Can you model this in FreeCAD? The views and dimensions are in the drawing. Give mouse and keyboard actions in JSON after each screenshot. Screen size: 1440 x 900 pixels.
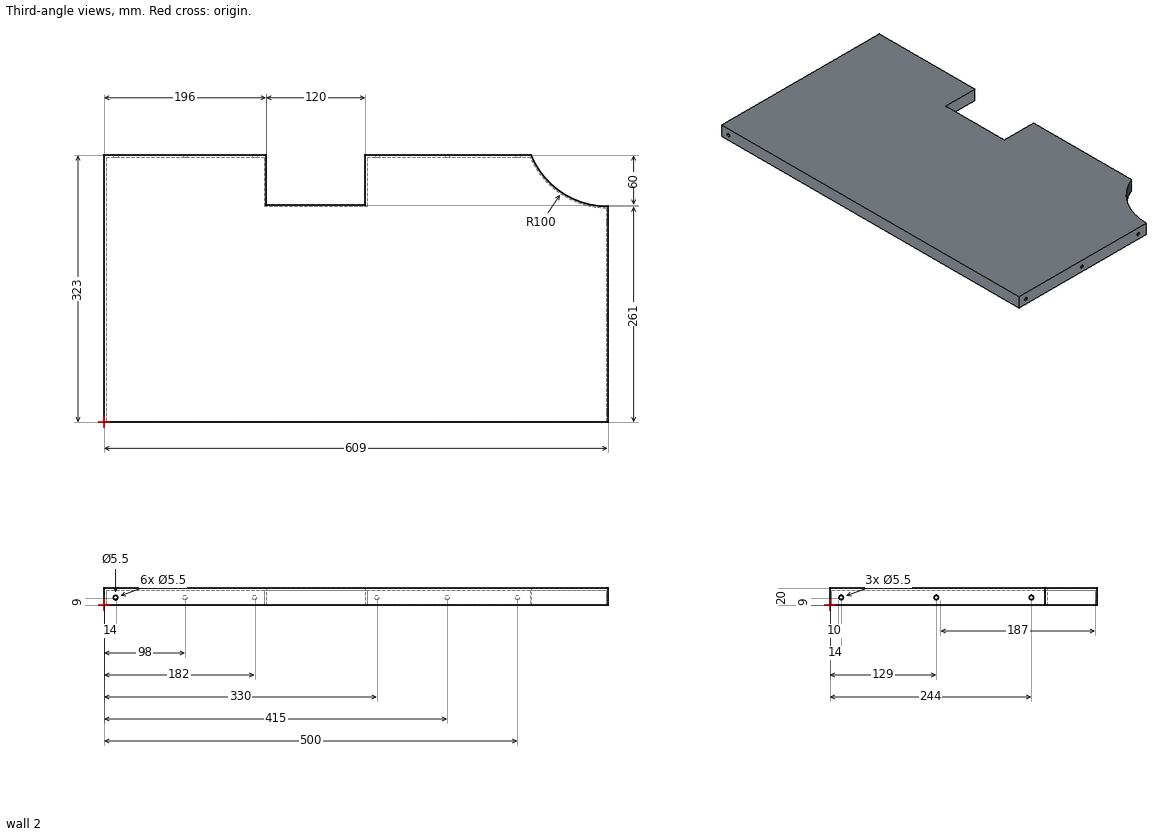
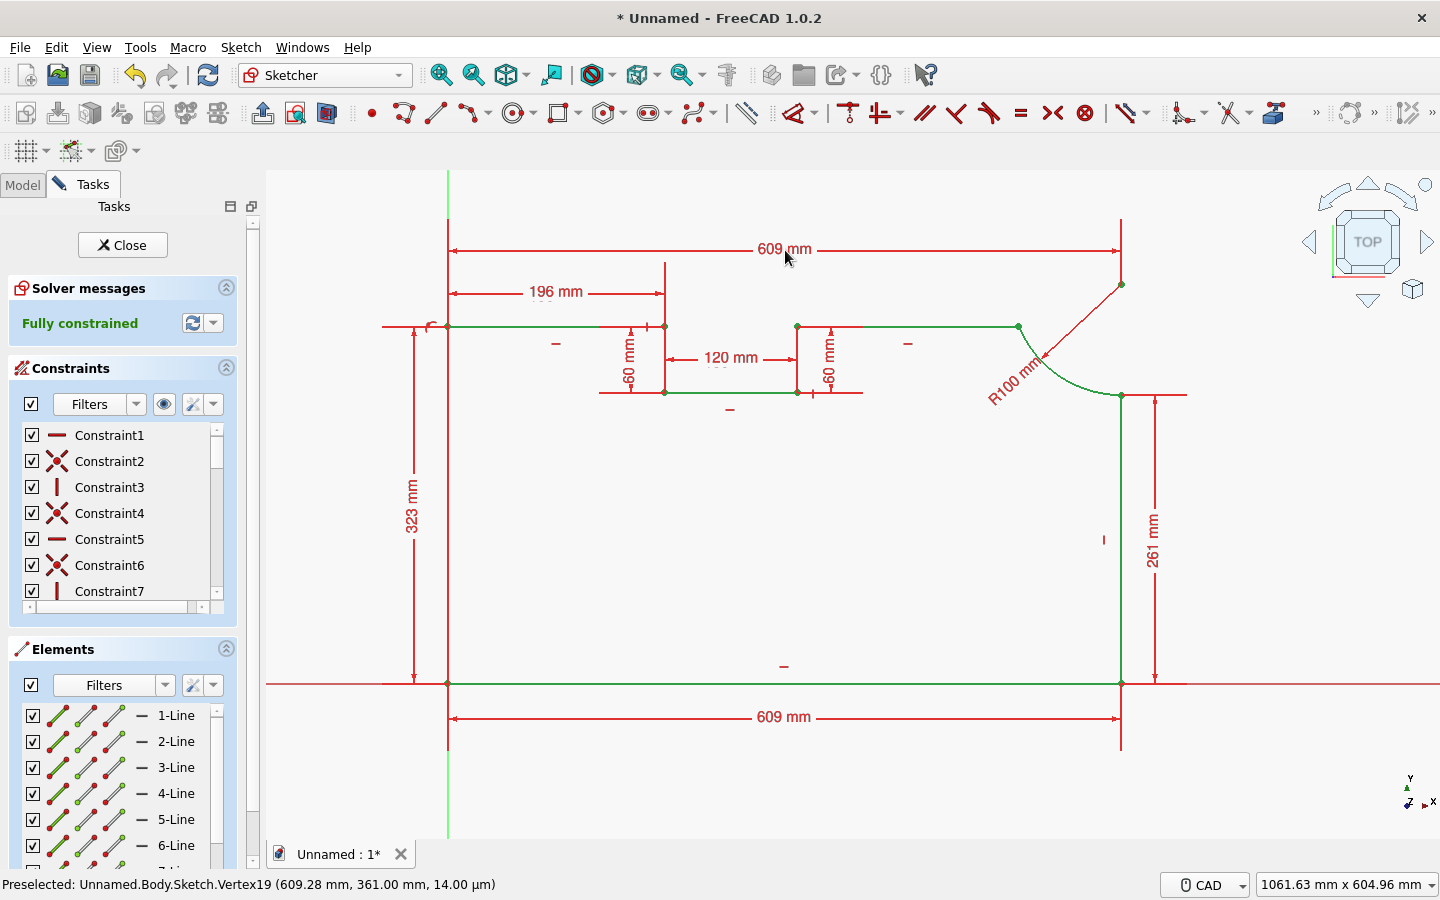
{"action": "left_click", "coordinate": [123, 245]}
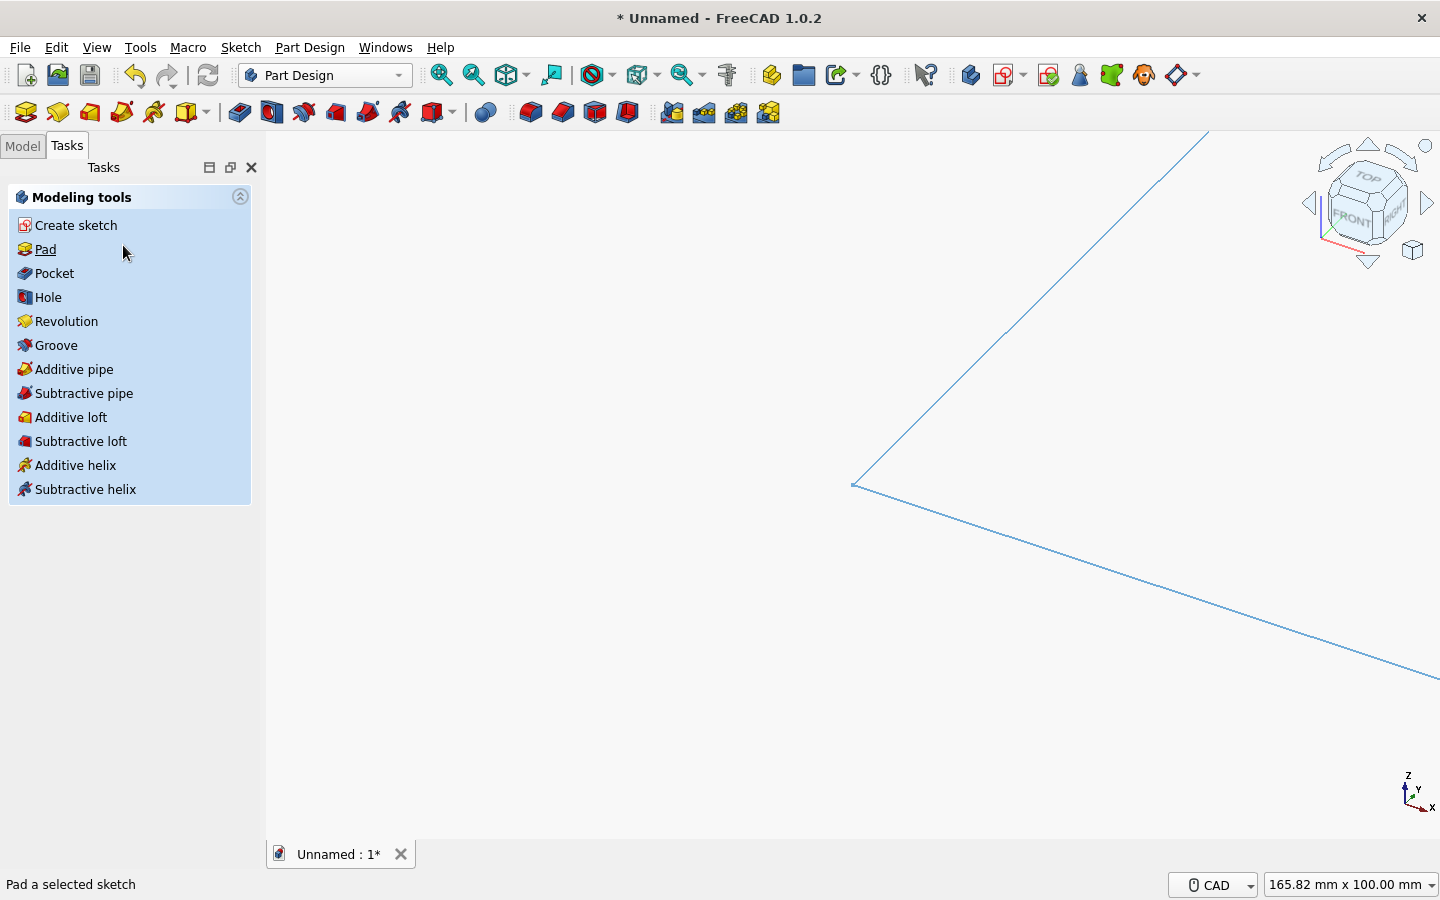
{"action": "left_click", "coordinate": [26, 112]}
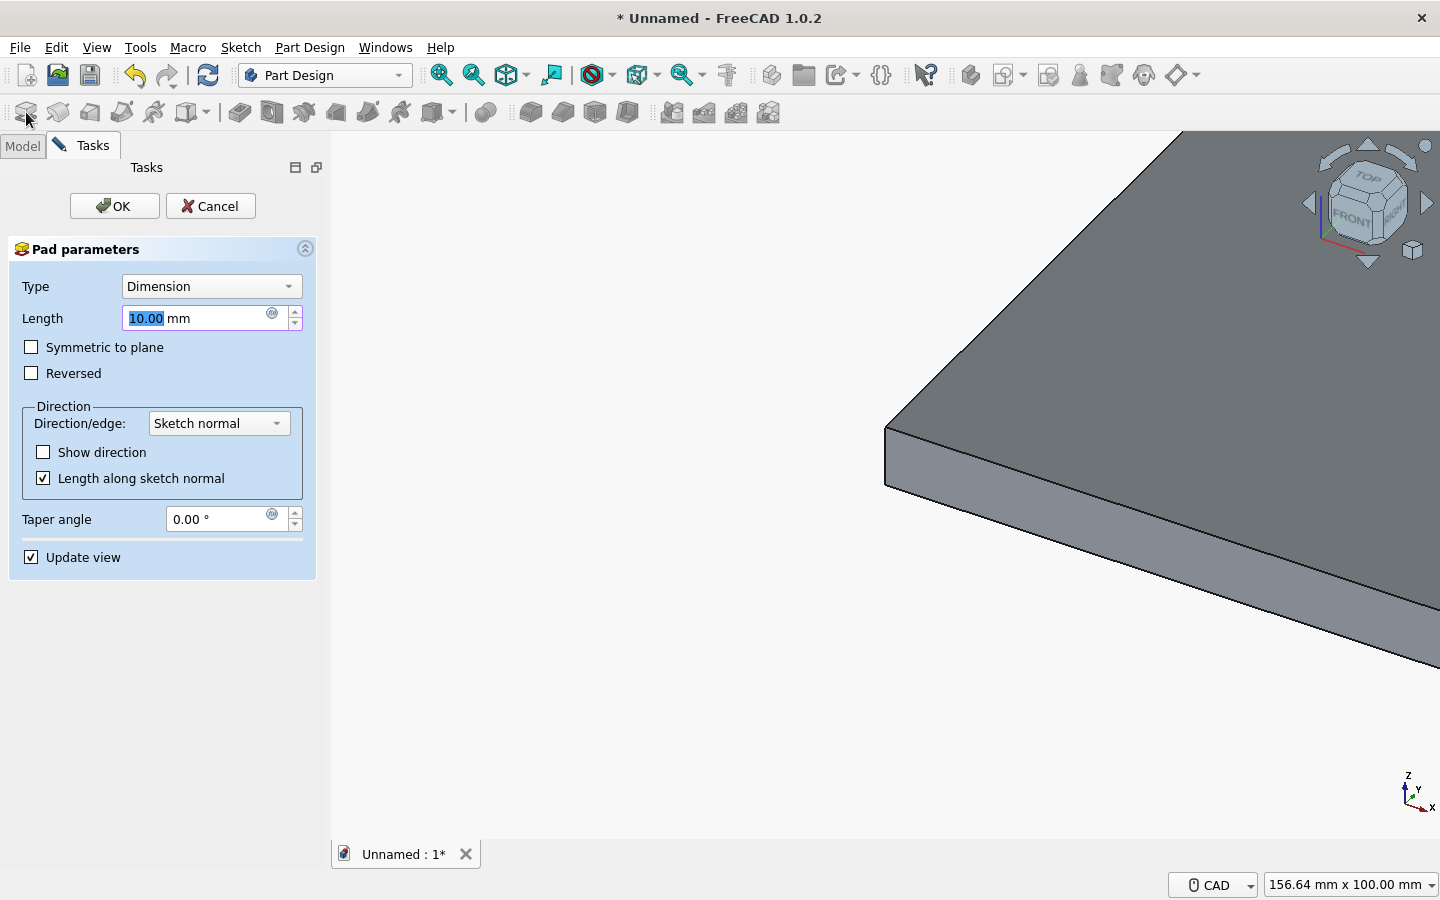
{"action": "type", "text": "20"}
{"action": "key", "text": "Tab"}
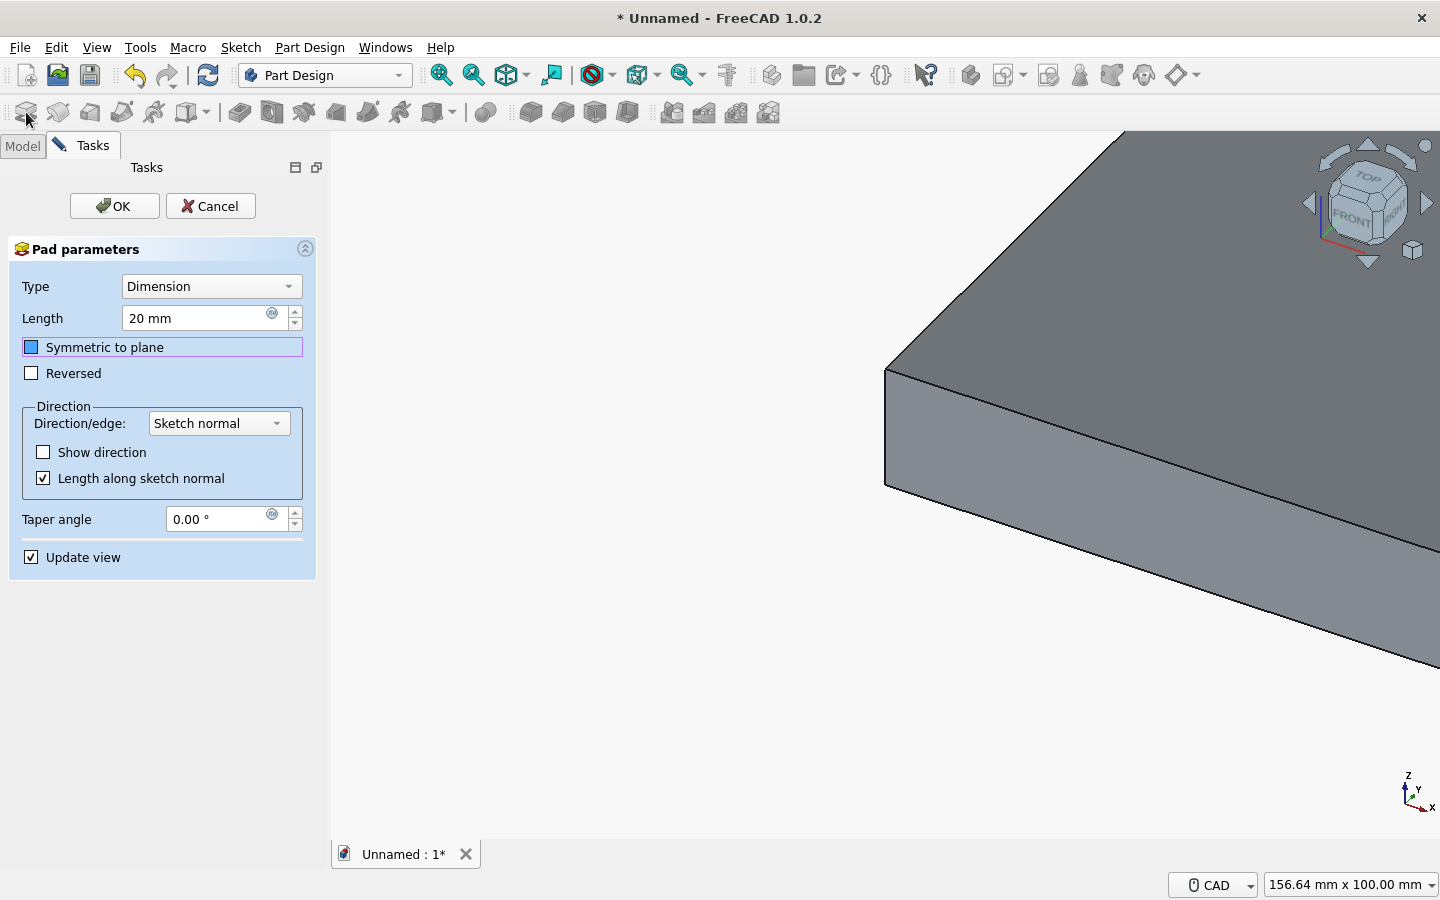
{"action": "left_click", "coordinate": [115, 206]}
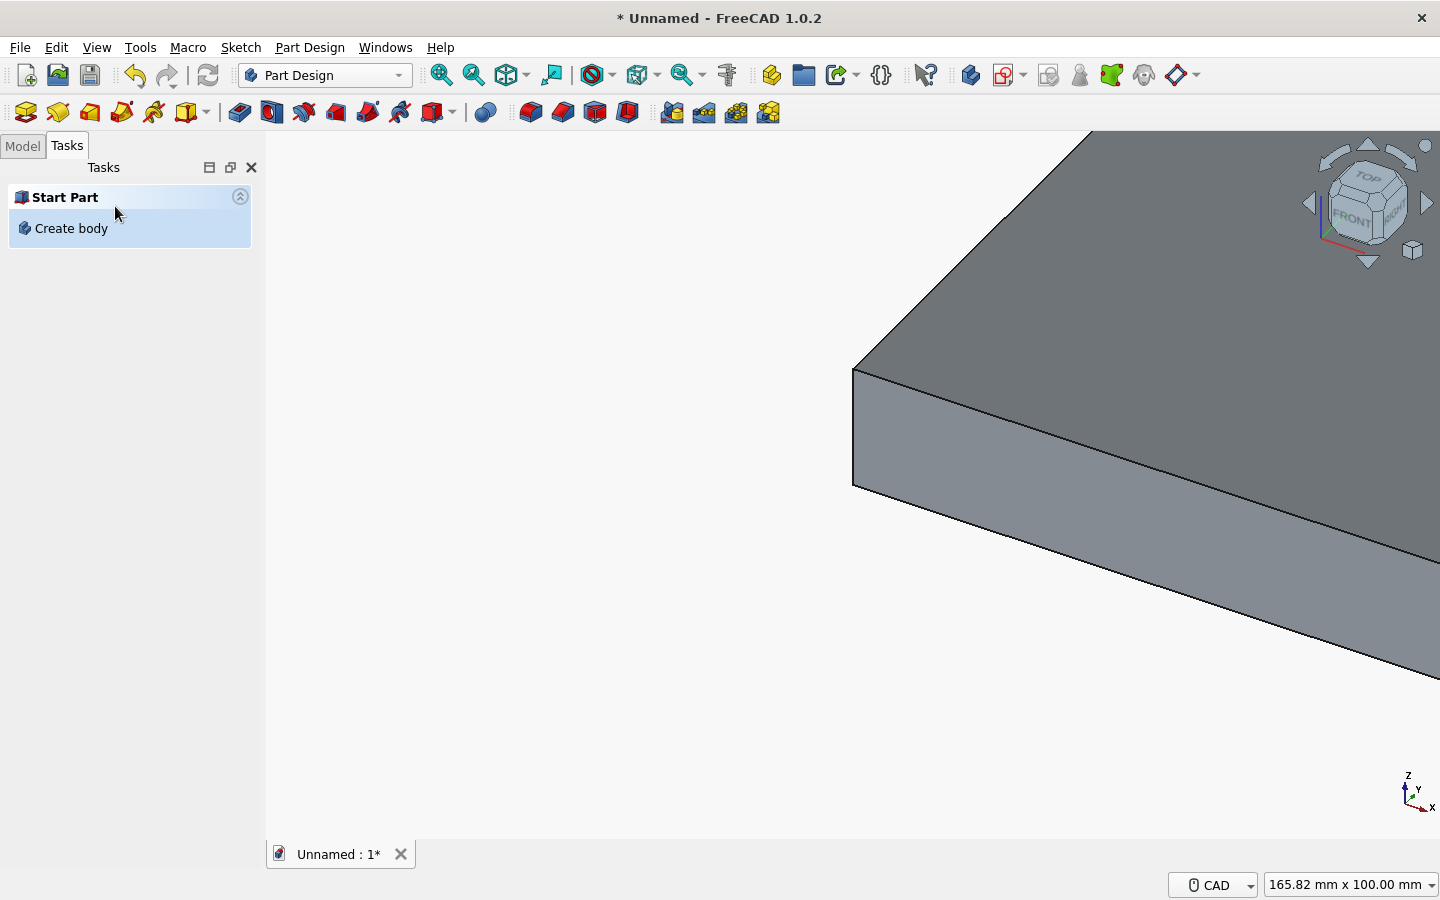
{"action": "left_click", "coordinate": [442, 76]}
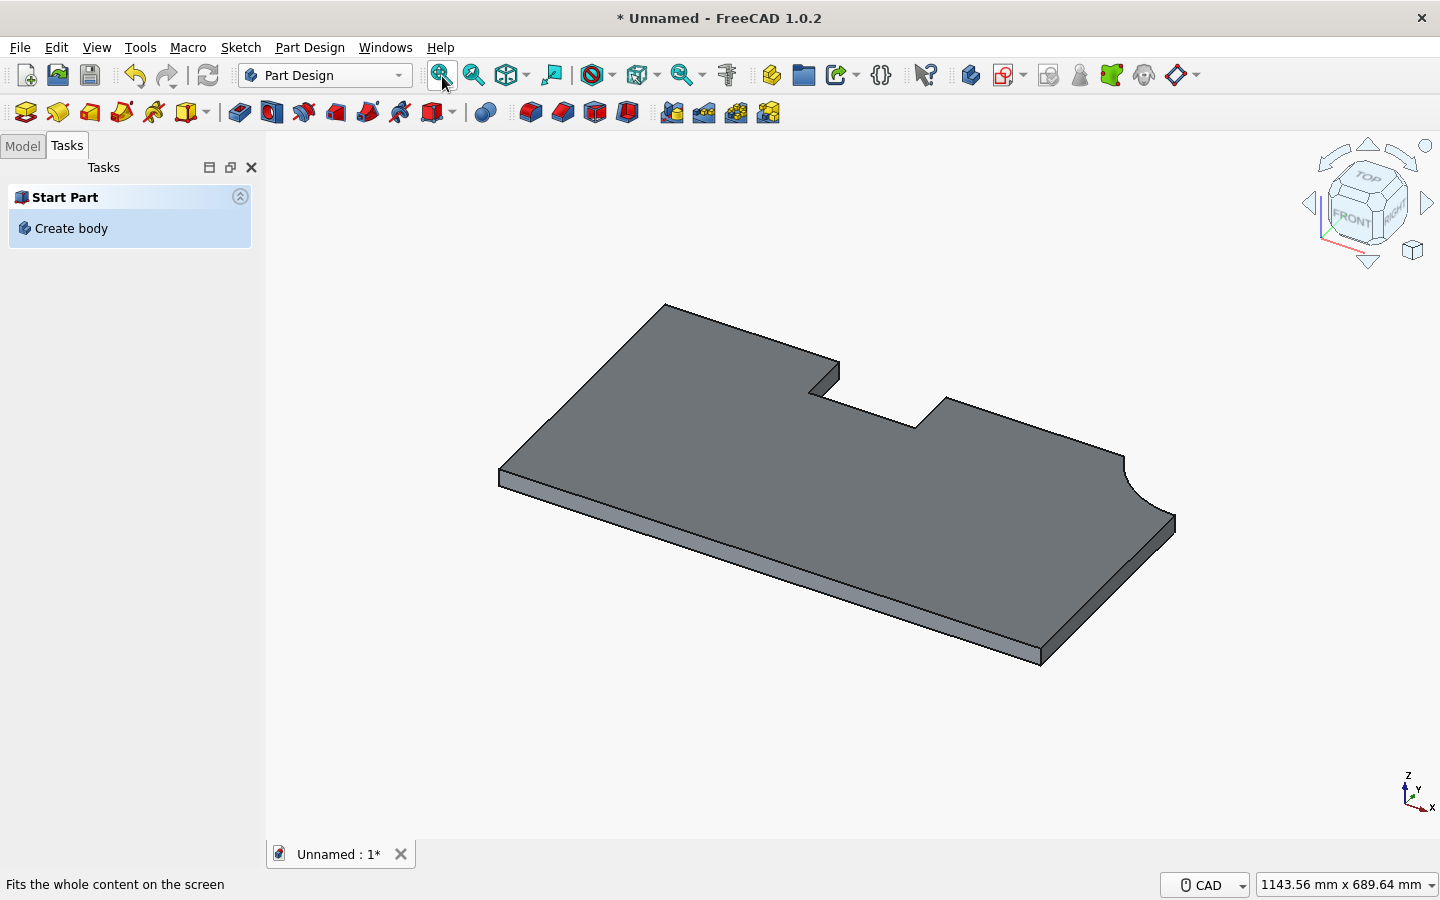
{"action": "key", "text": "0"}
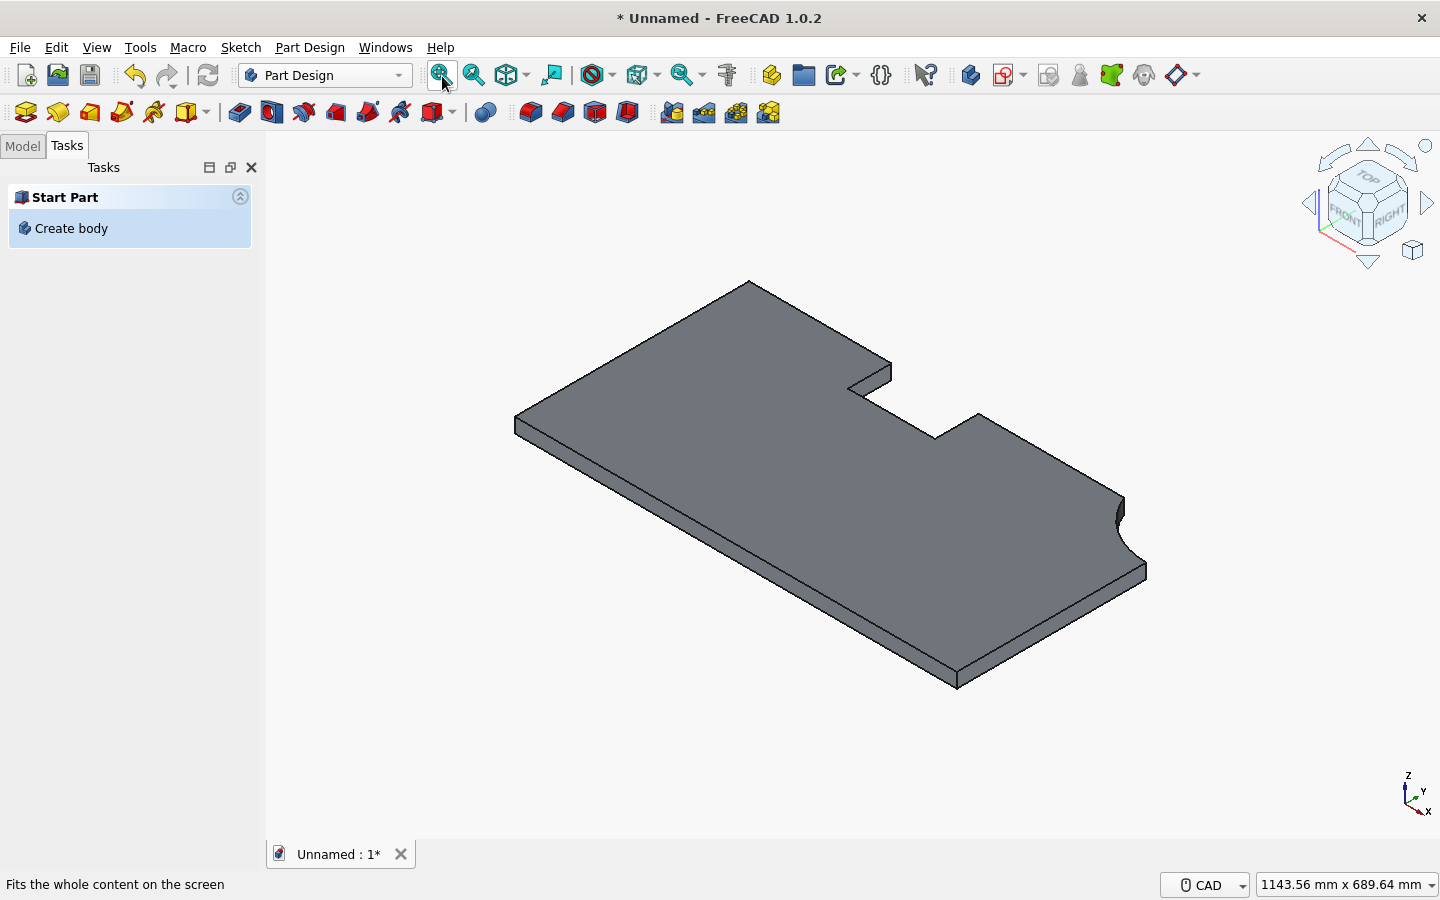
{"action": "key", "text": "2"}